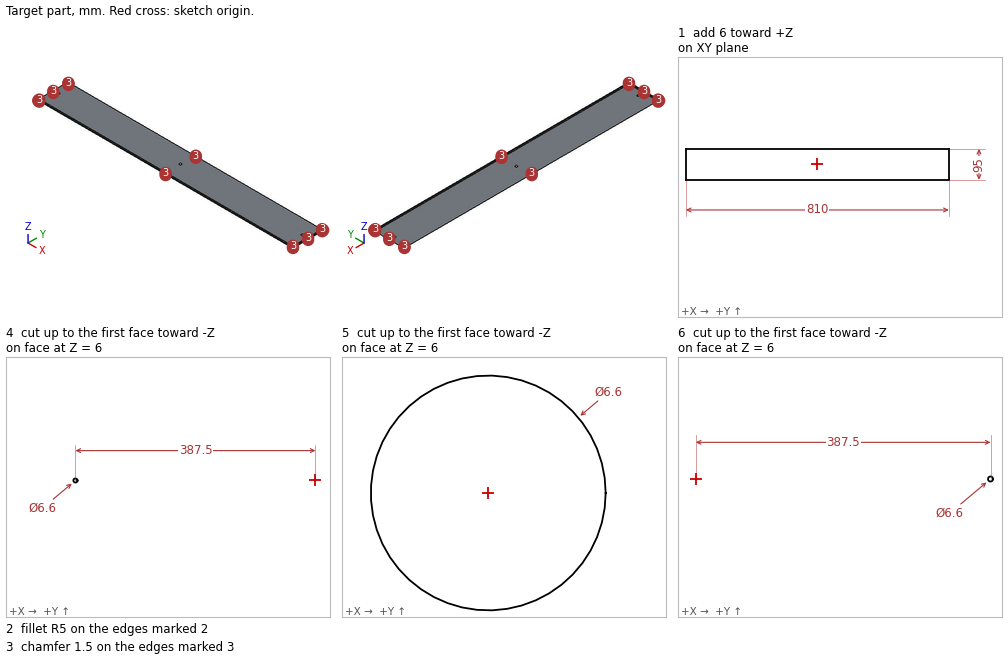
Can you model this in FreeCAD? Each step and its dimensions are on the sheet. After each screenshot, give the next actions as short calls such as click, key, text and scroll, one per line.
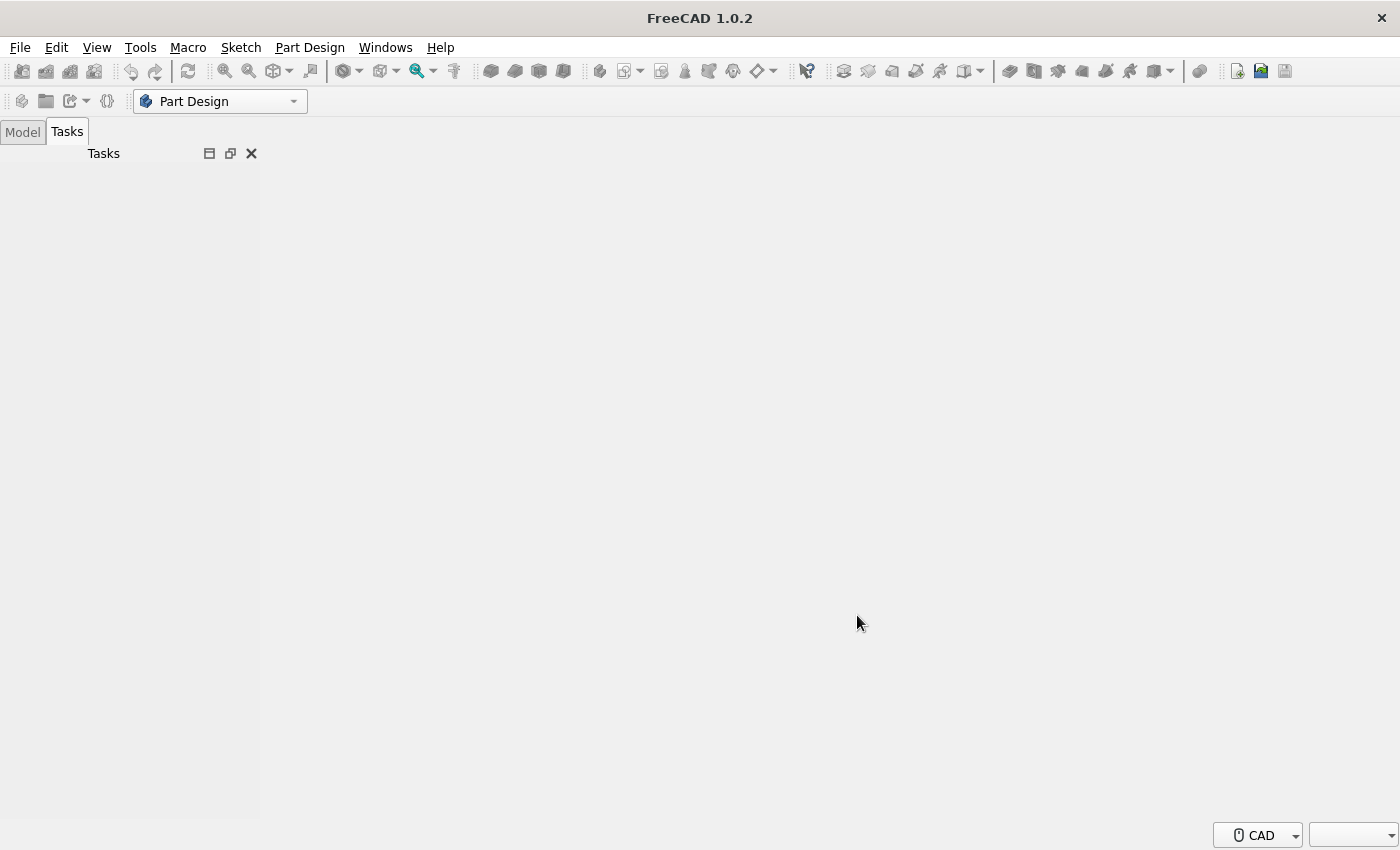
key(ctrl+n)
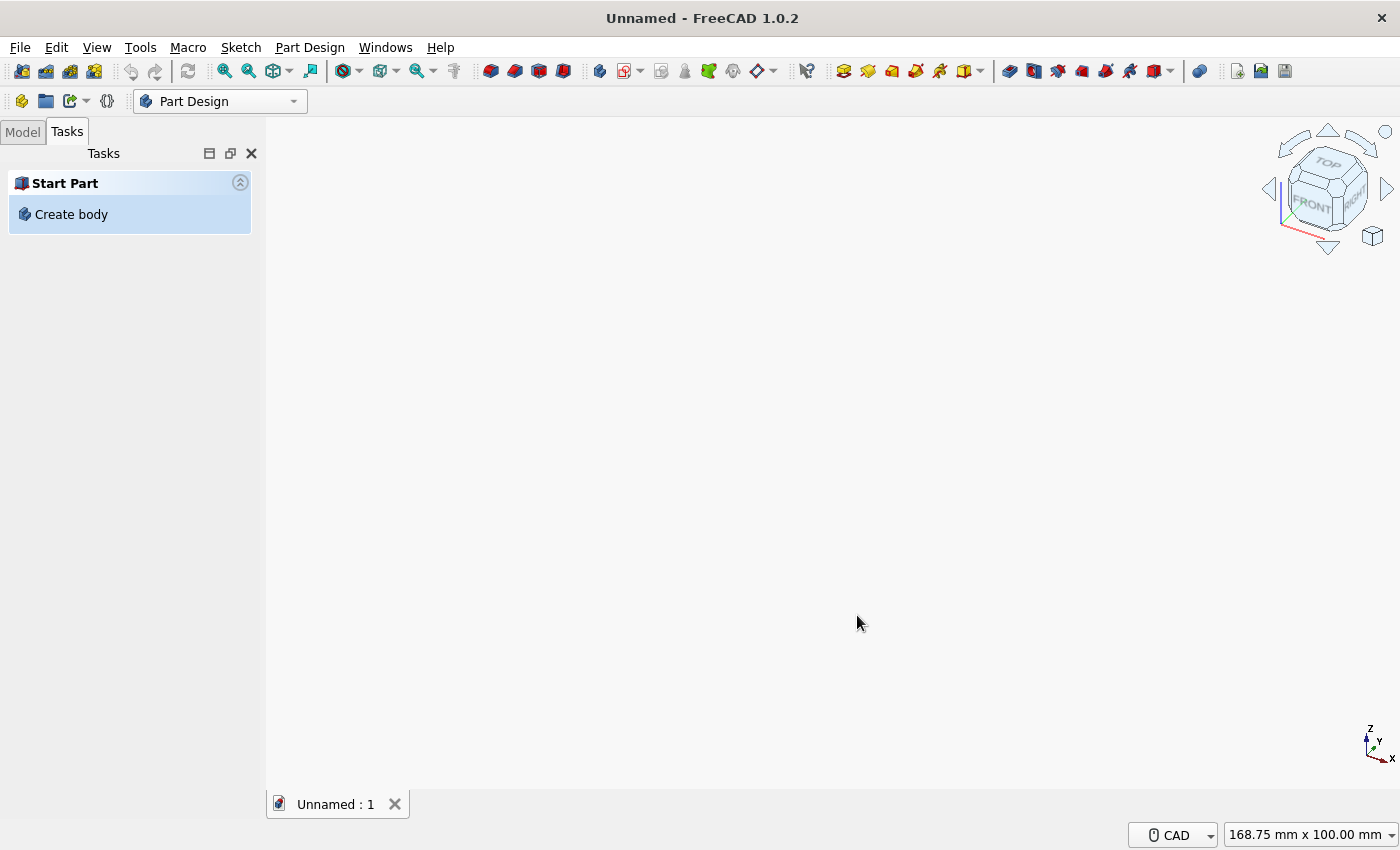
click(624, 72)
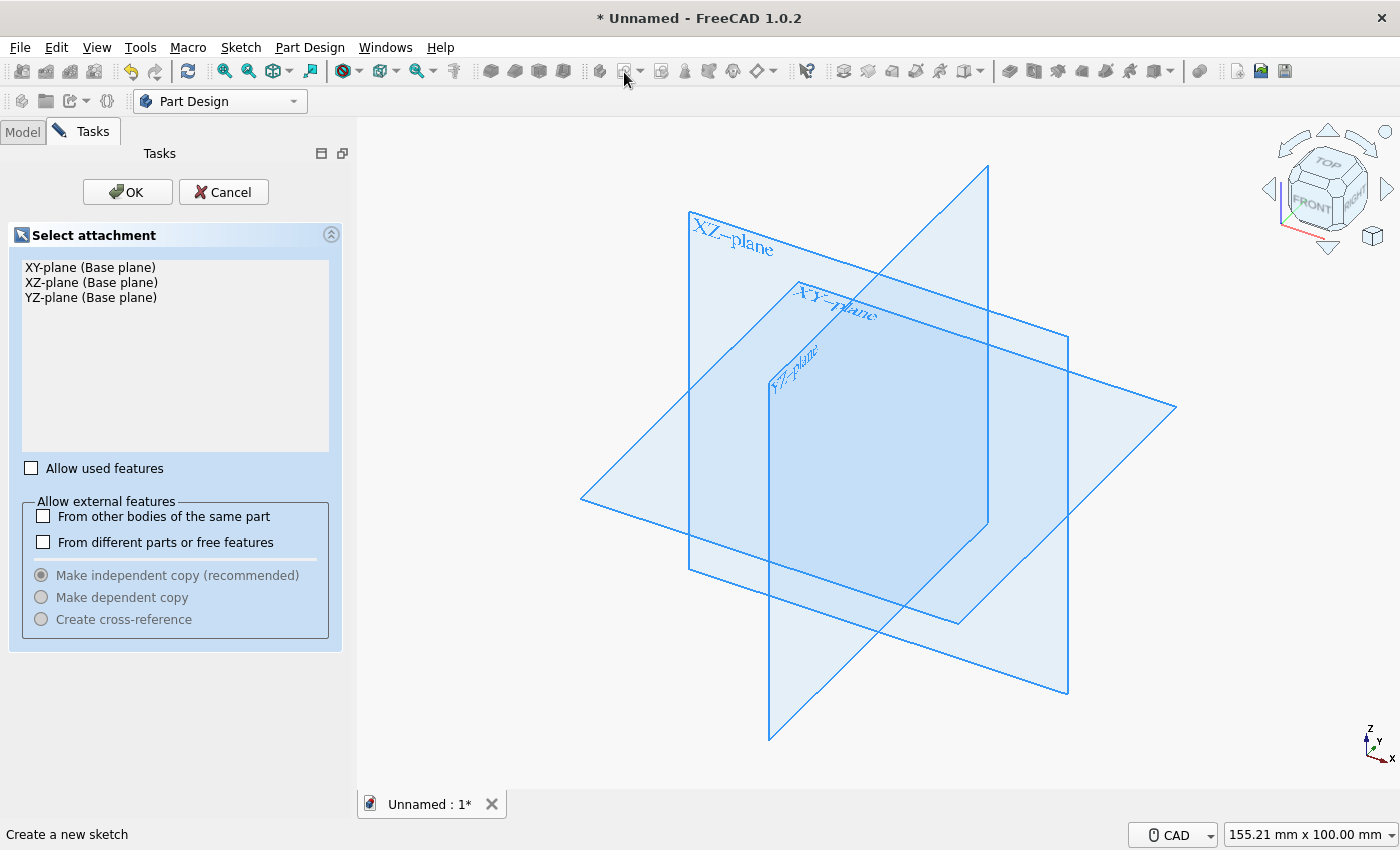
click(82, 268)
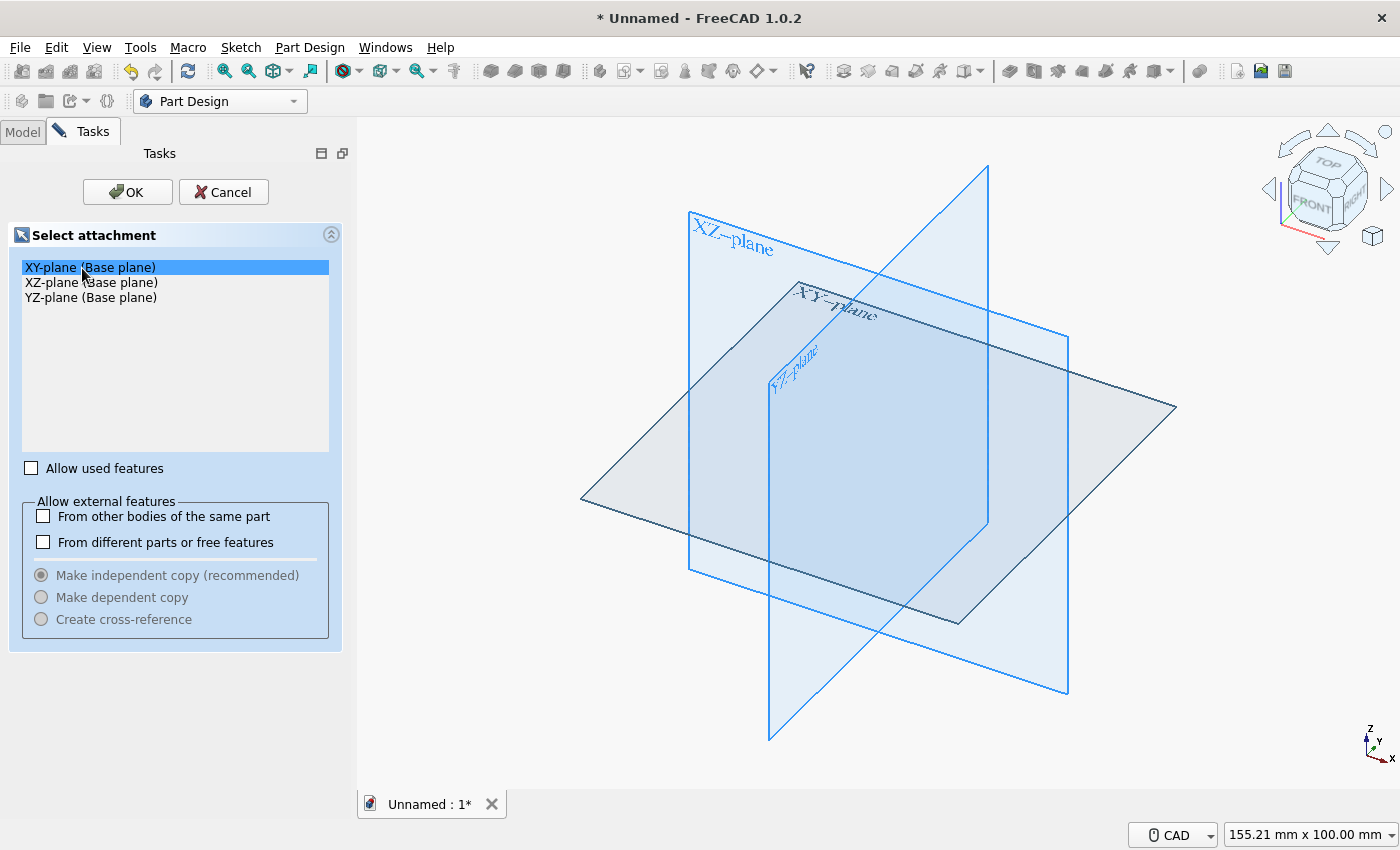
click(128, 192)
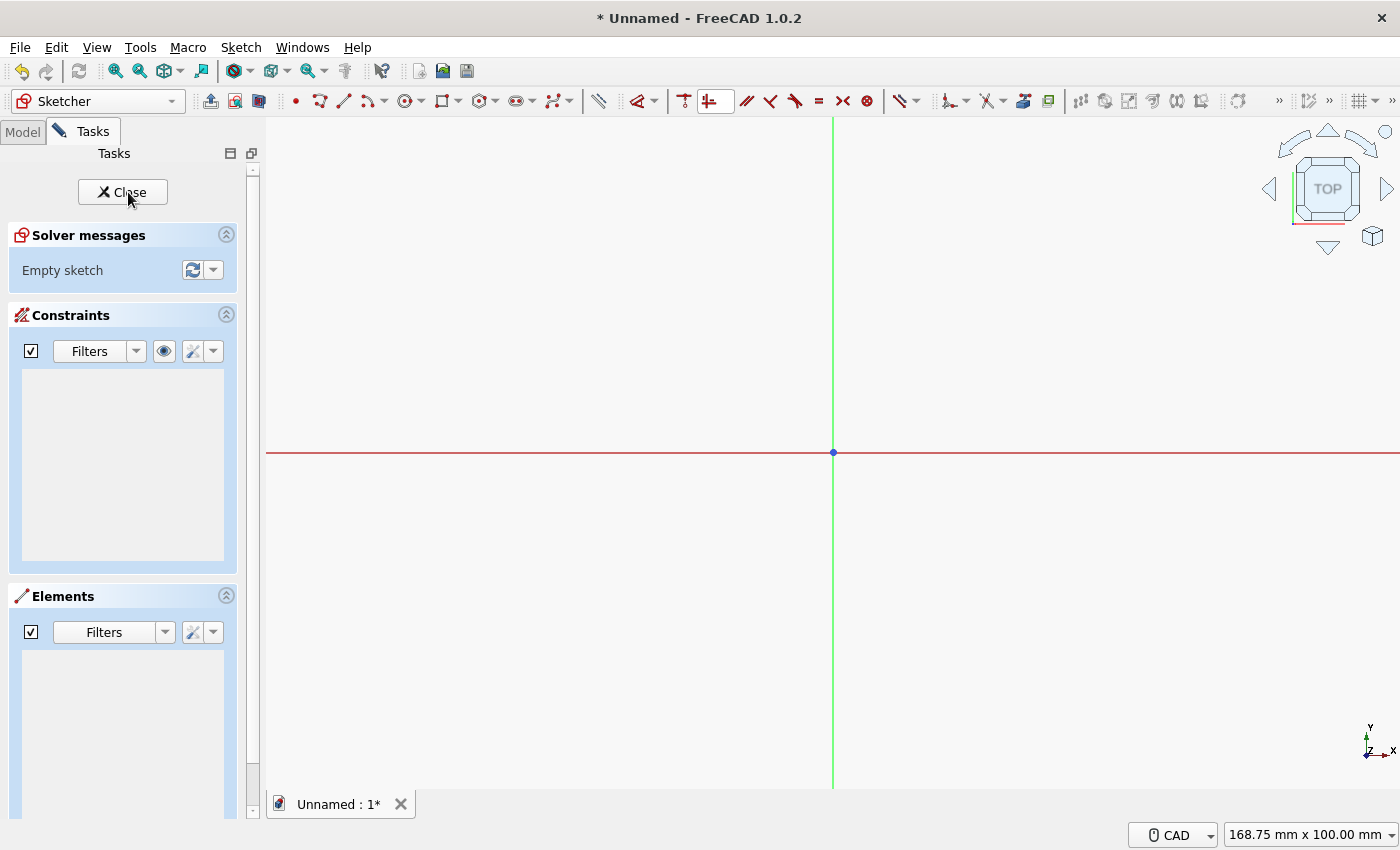
scroll(756, 453, down, 11)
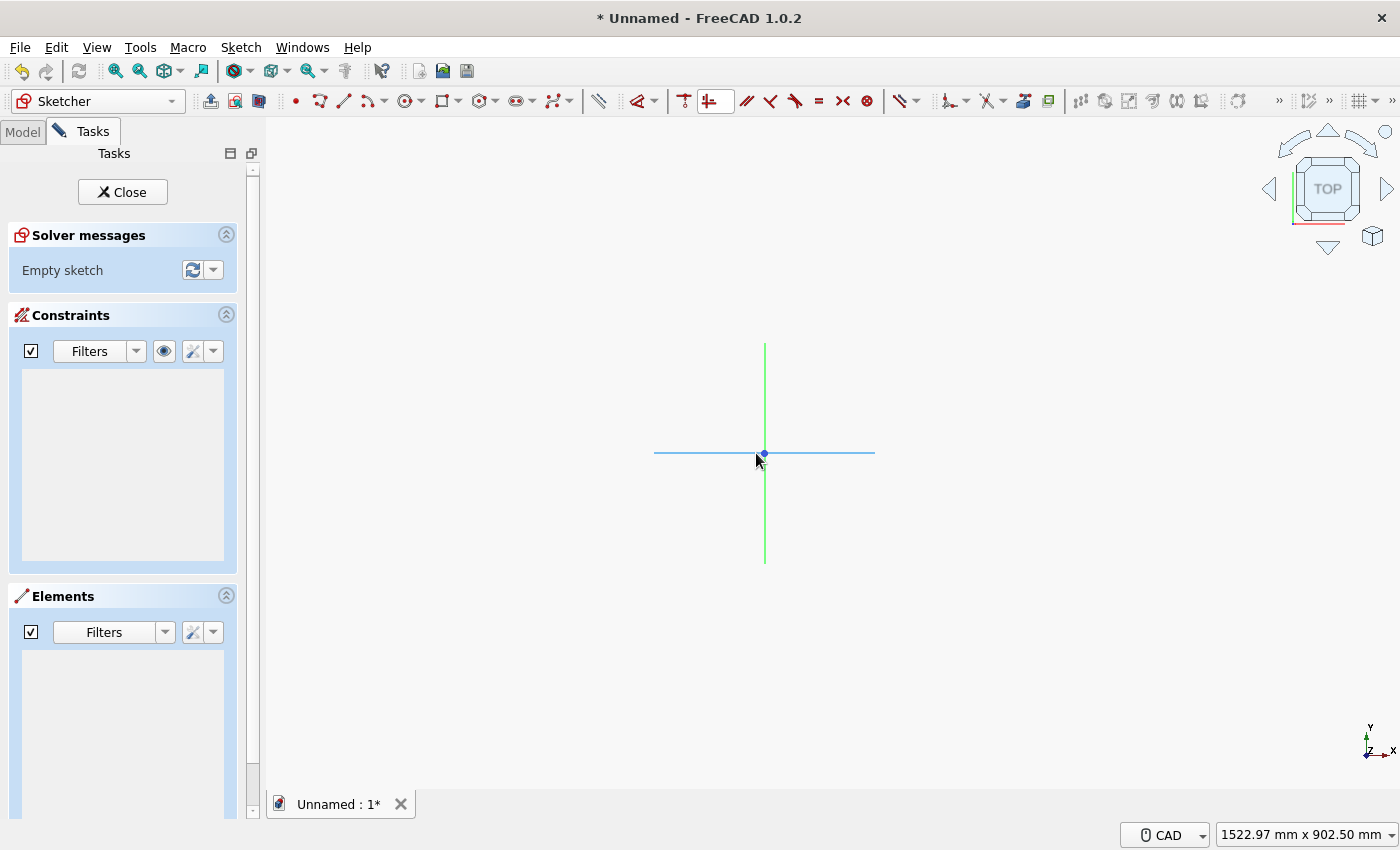
key(g)
key(v)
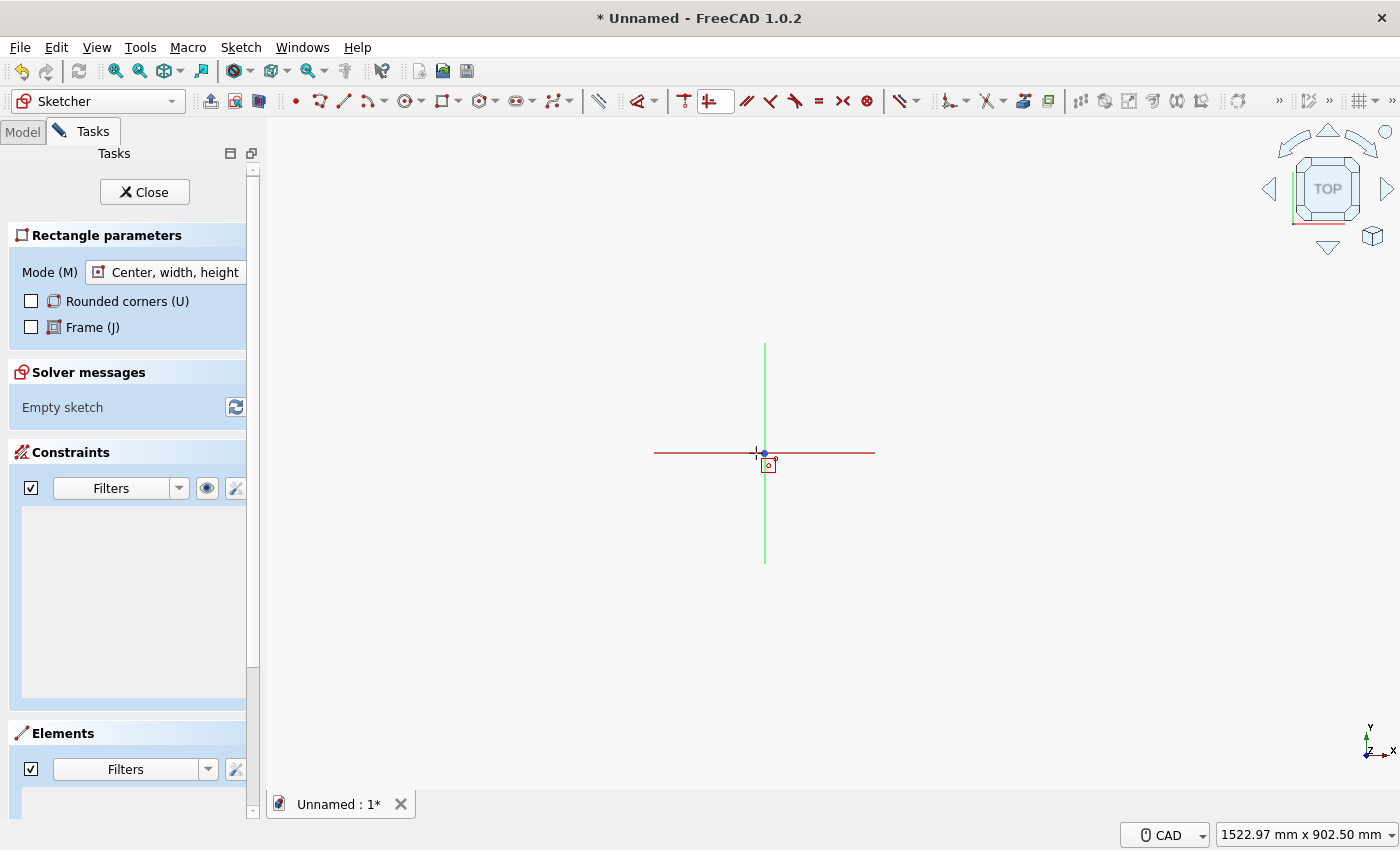
click(765, 453)
move(1066, 418)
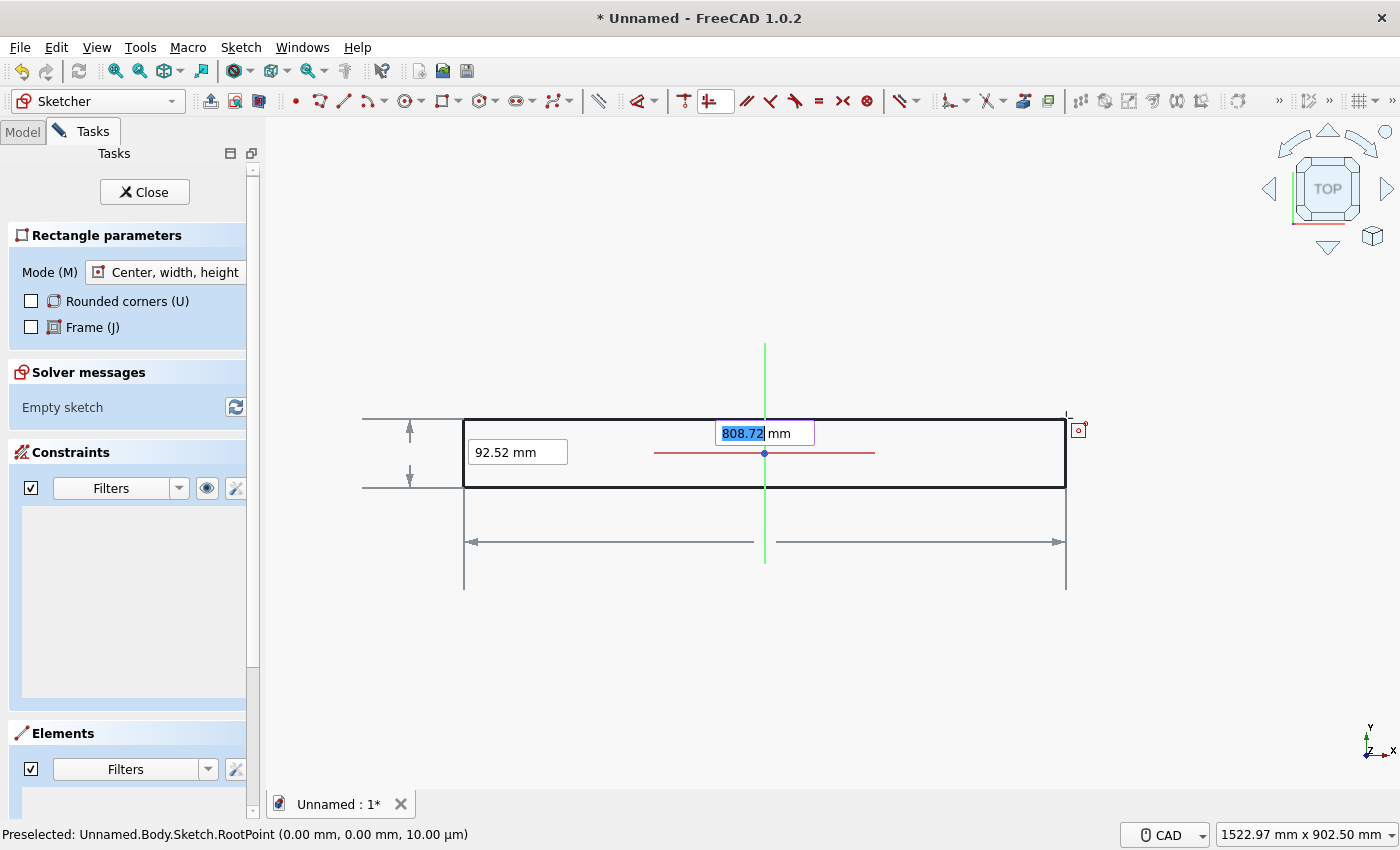
text(810)
key(Tab)
text(95)
key(Return)
key(Escape)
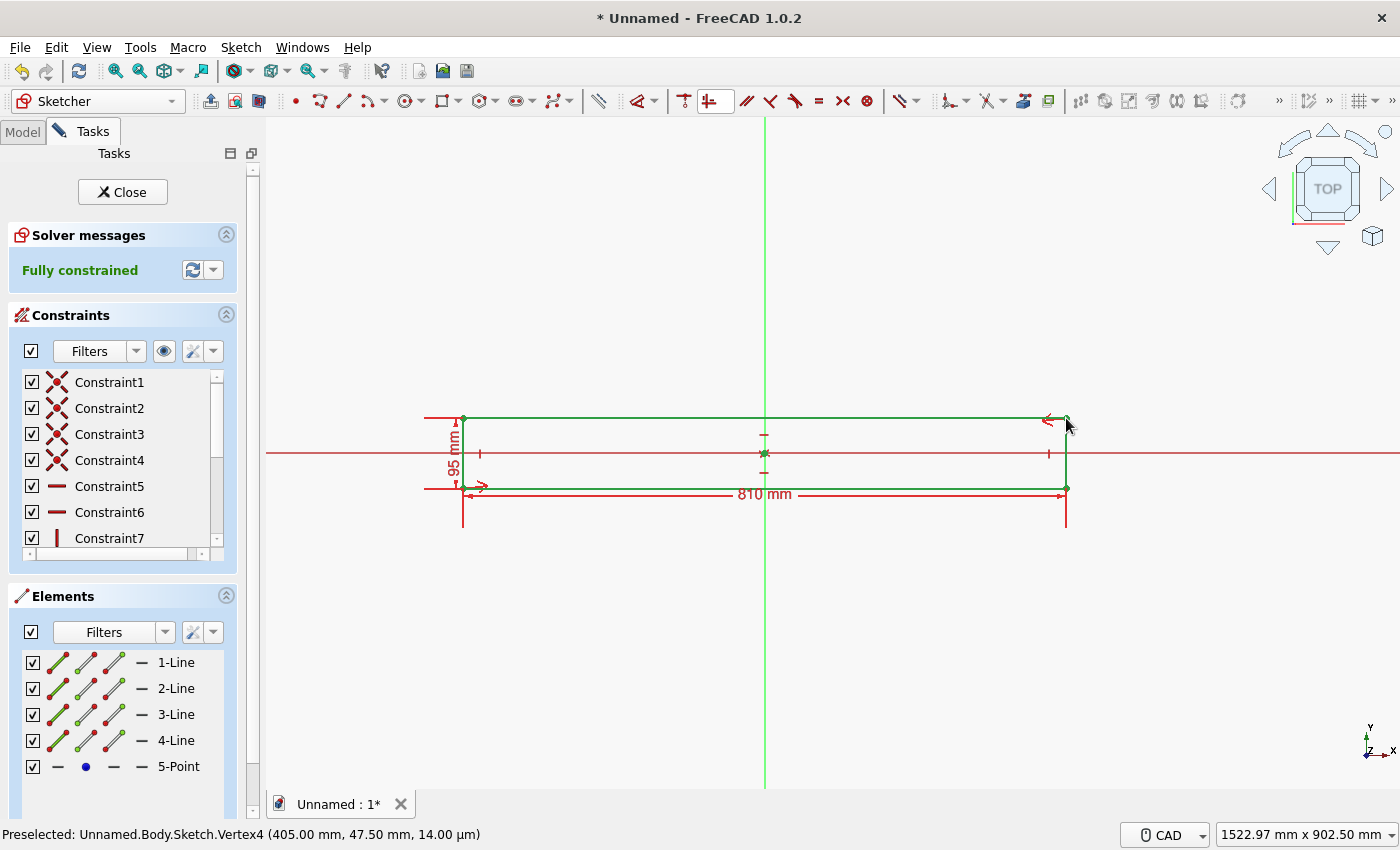
click(123, 192)